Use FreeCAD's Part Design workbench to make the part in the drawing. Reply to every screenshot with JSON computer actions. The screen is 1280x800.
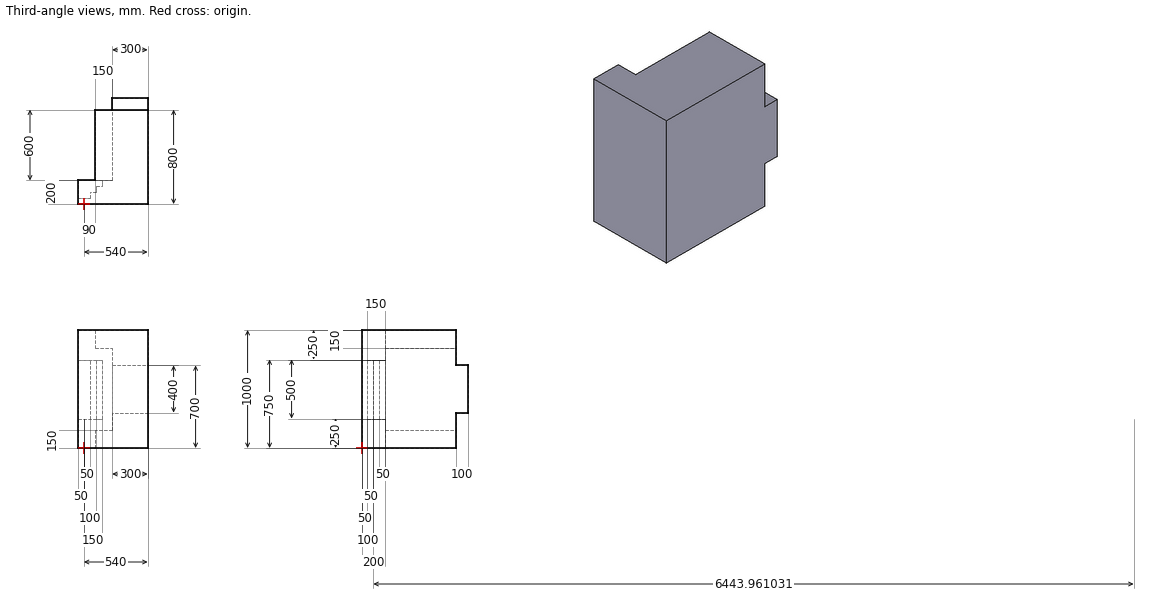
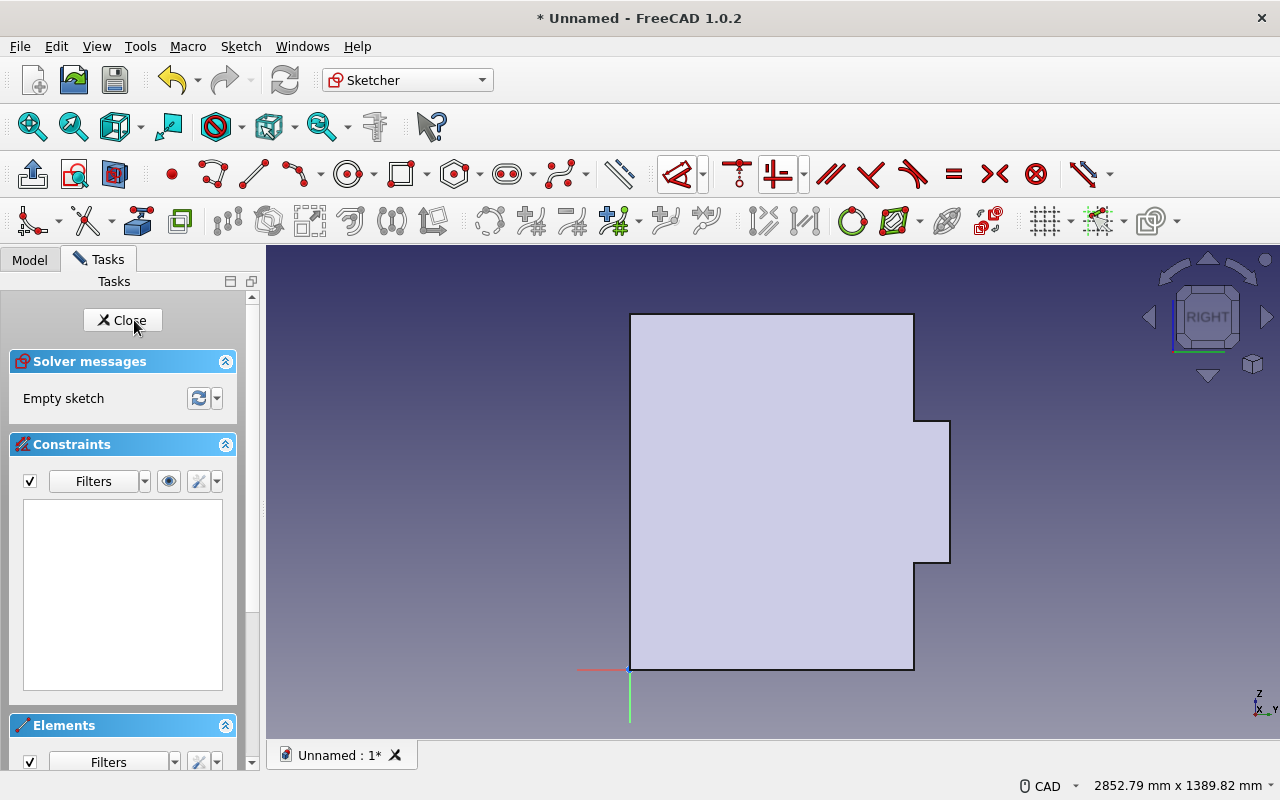
{"action": "left_click", "coordinate": [115, 174]}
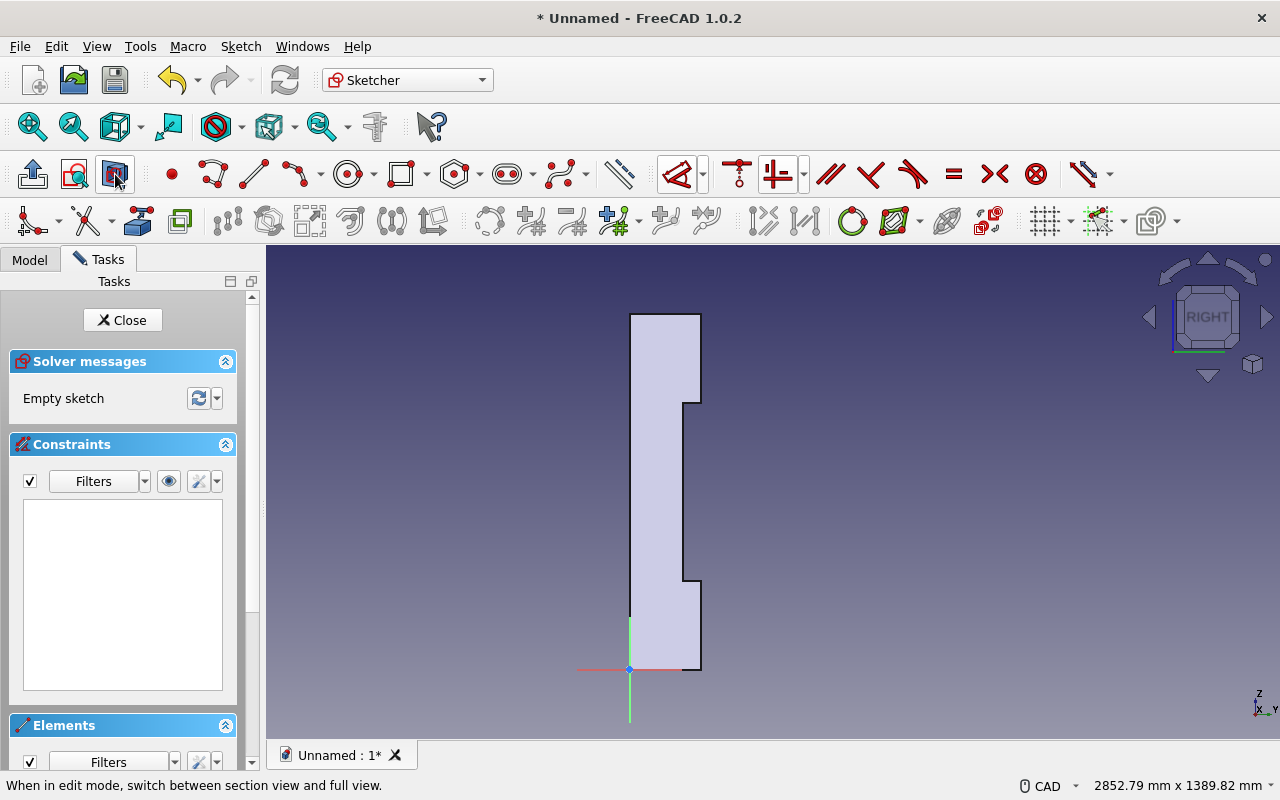
{"action": "scroll", "coordinate": [348, 477], "scroll_direction": "down", "scroll_amount": 7}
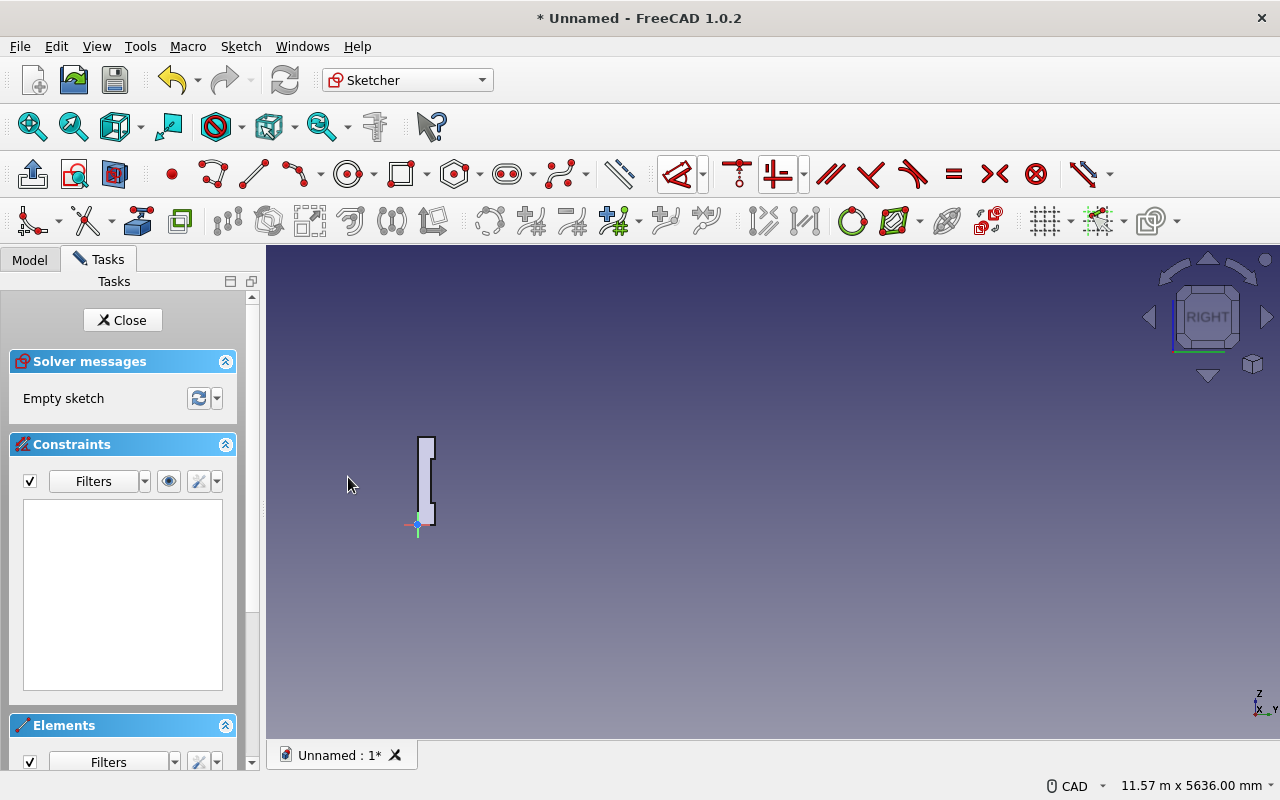
{"action": "left_click", "coordinate": [400, 174]}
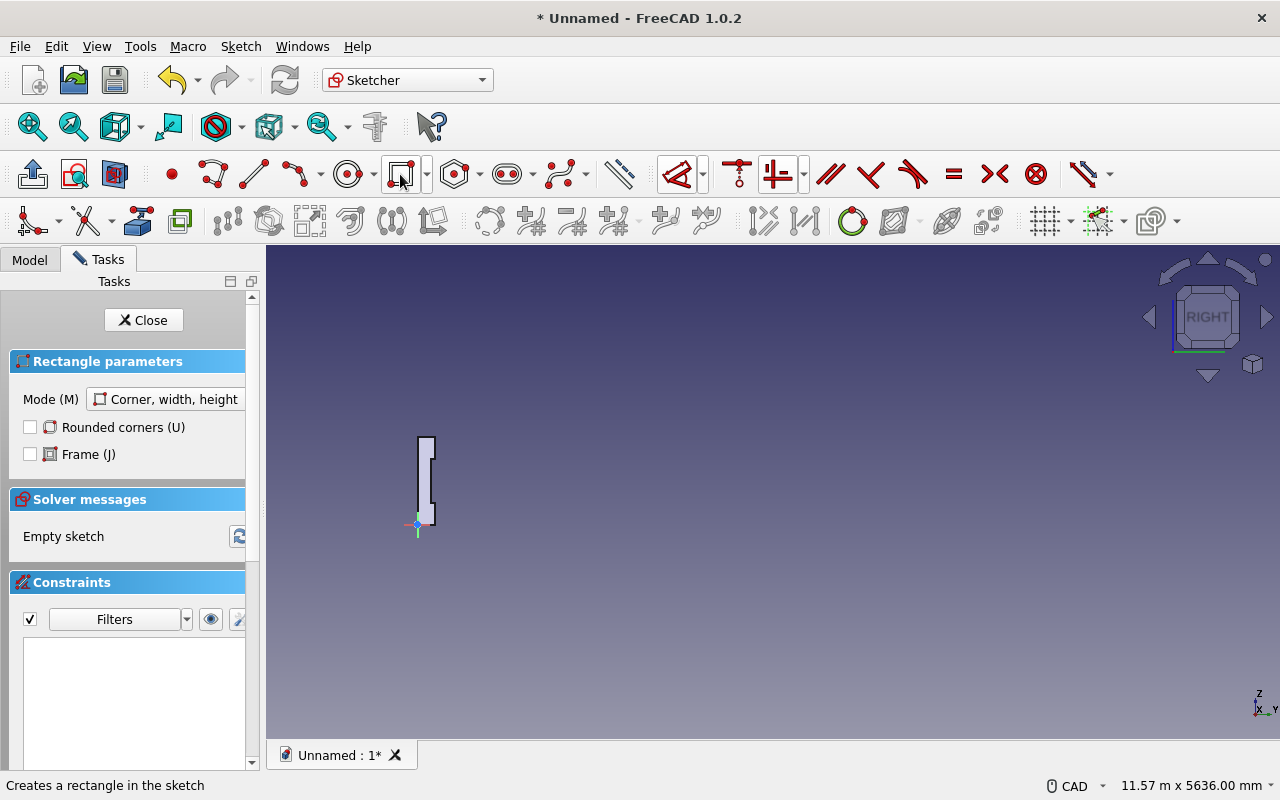
{"action": "scroll", "coordinate": [426, 459], "scroll_direction": "up", "scroll_amount": 3}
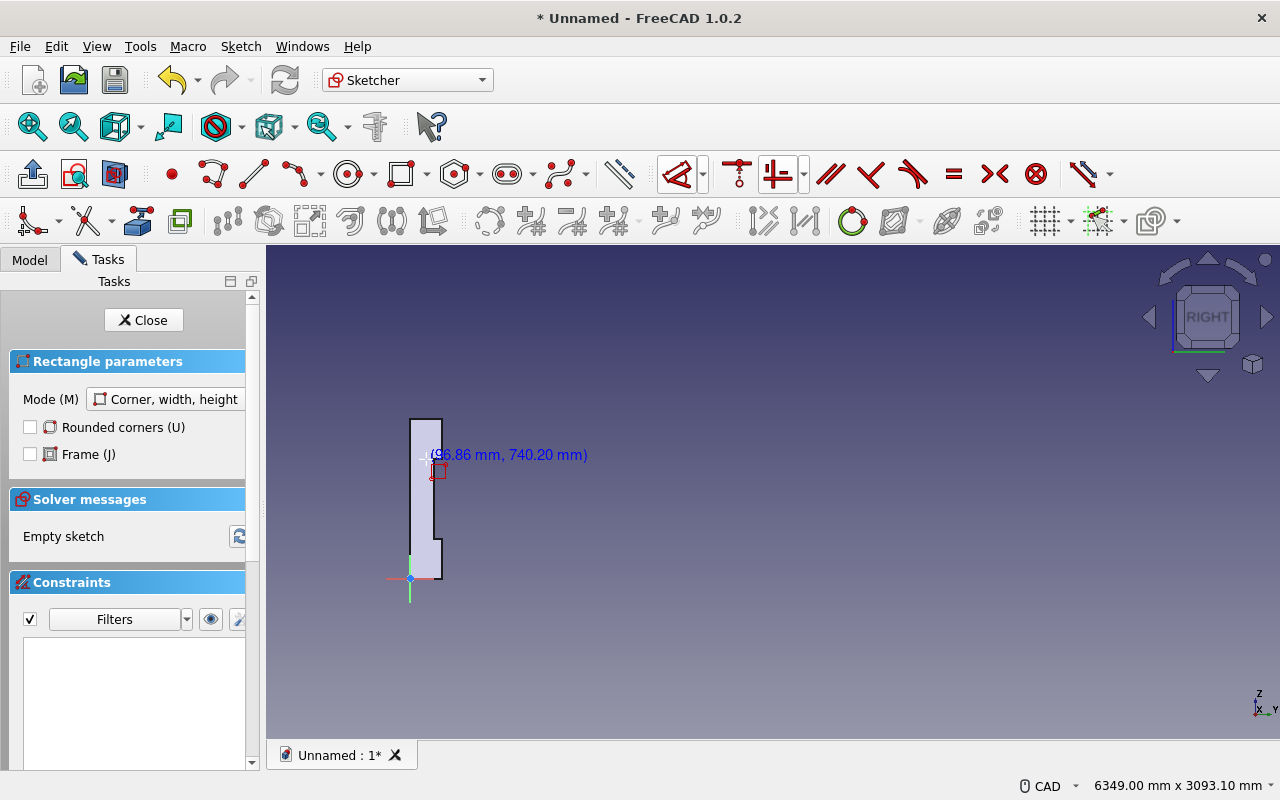
{"action": "left_click", "coordinate": [426, 459]}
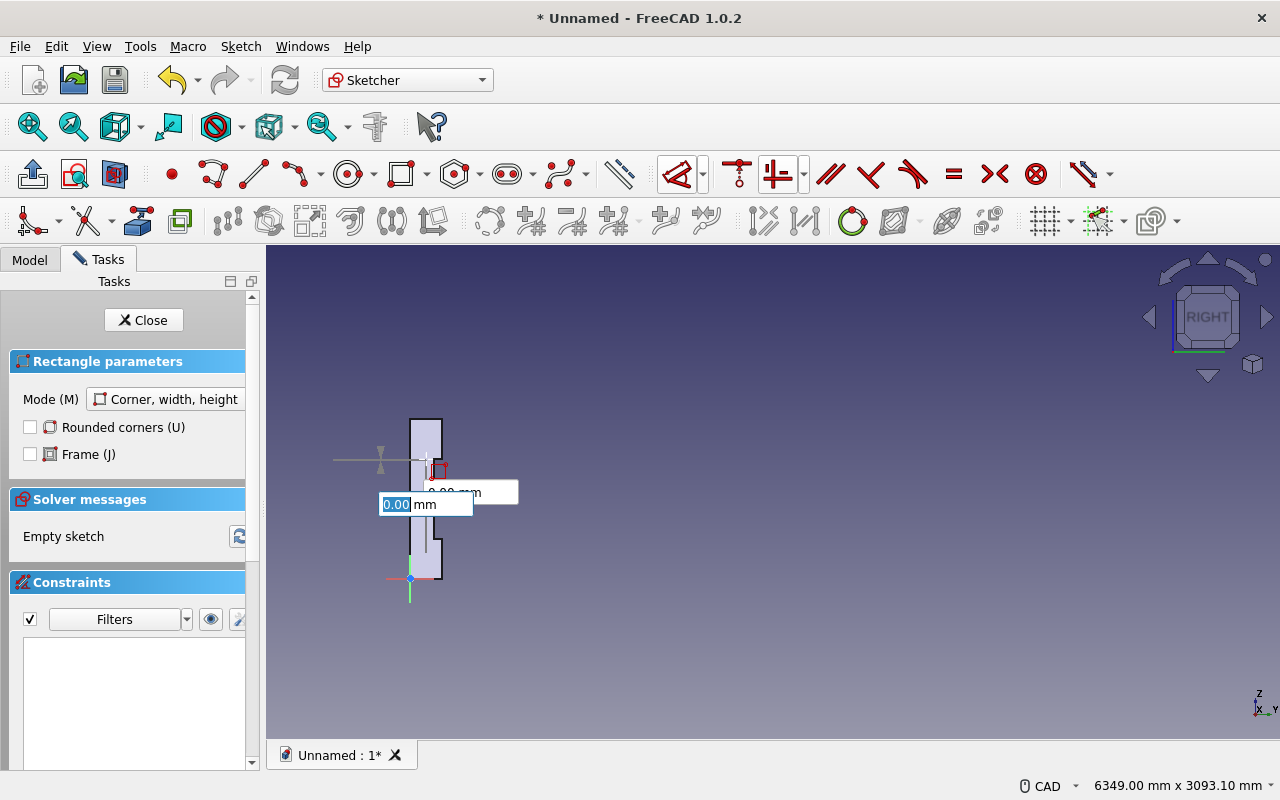
{"action": "scroll", "coordinate": [427, 459], "scroll_direction": "down", "scroll_amount": 3}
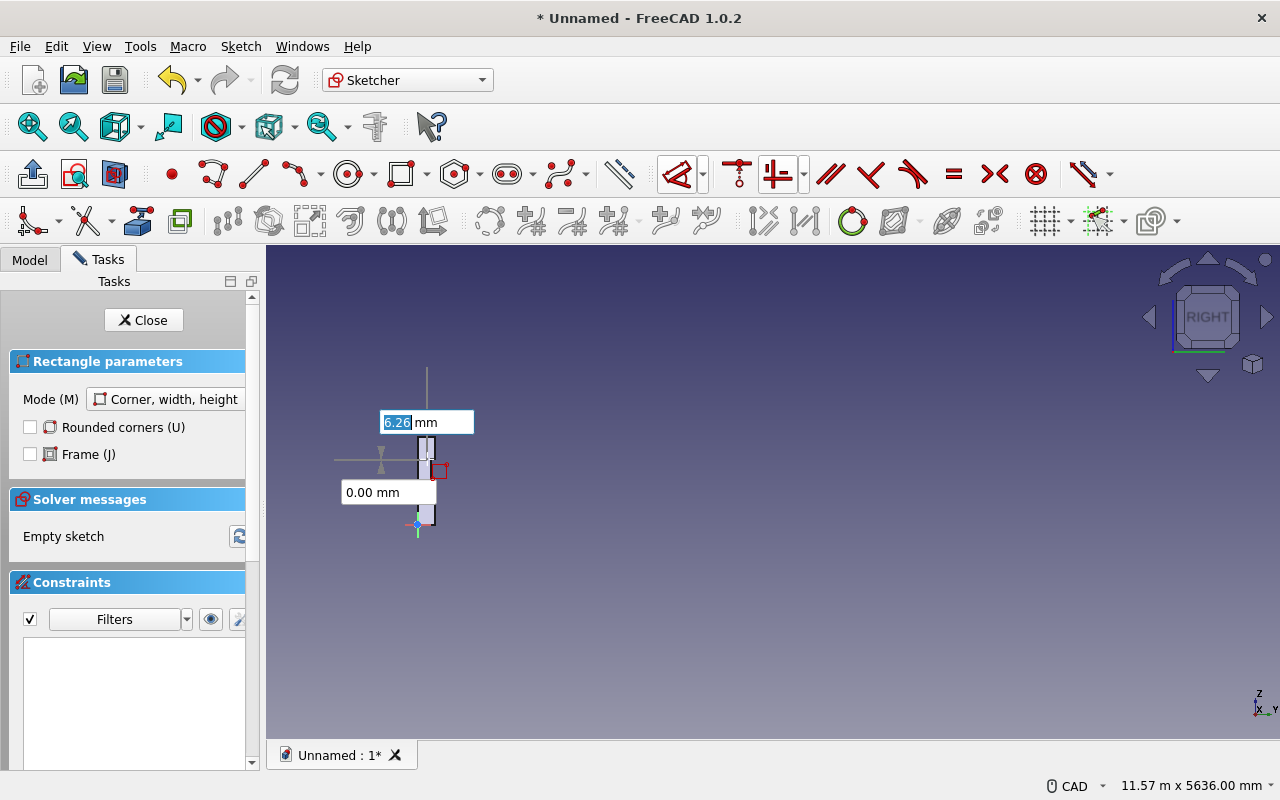
{"action": "left_click", "coordinate": [992, 503]}
{"action": "key", "text": "Escape"}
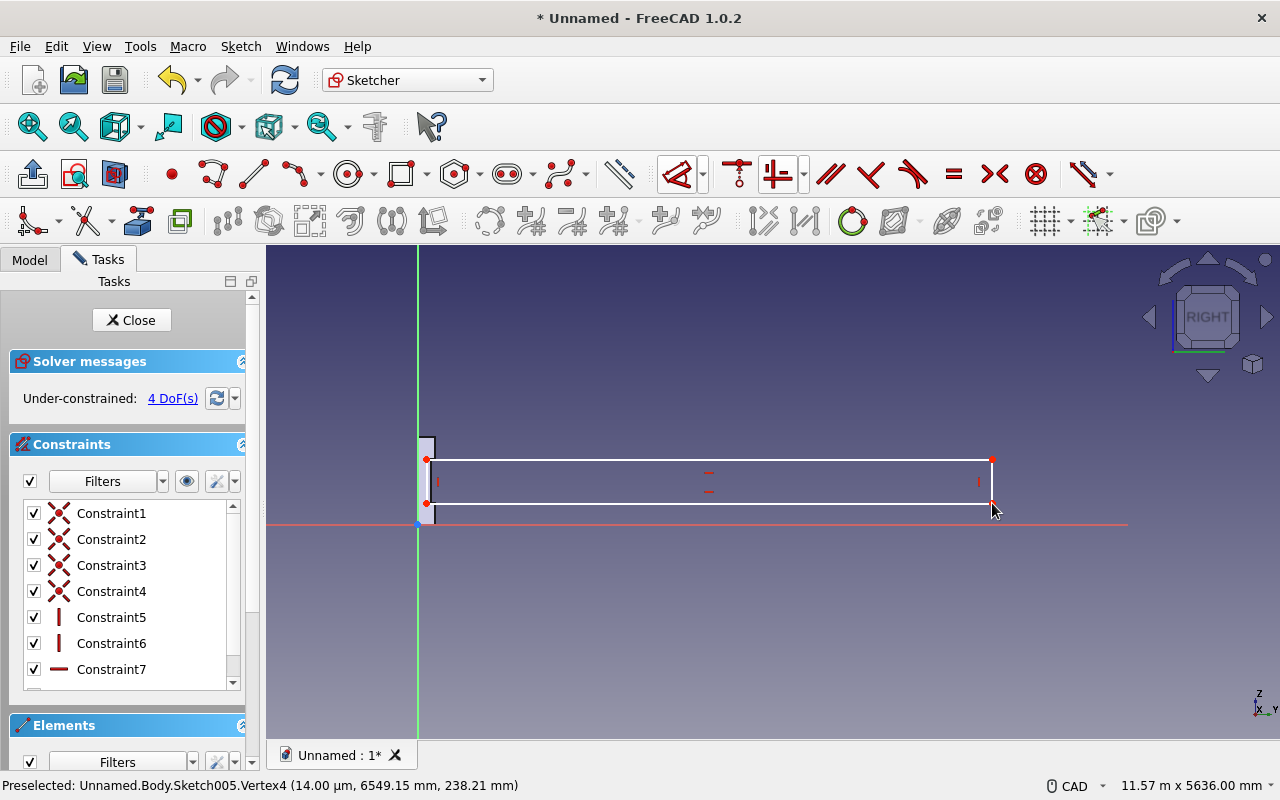
{"action": "scroll", "coordinate": [427, 473], "scroll_direction": "up", "scroll_amount": 3}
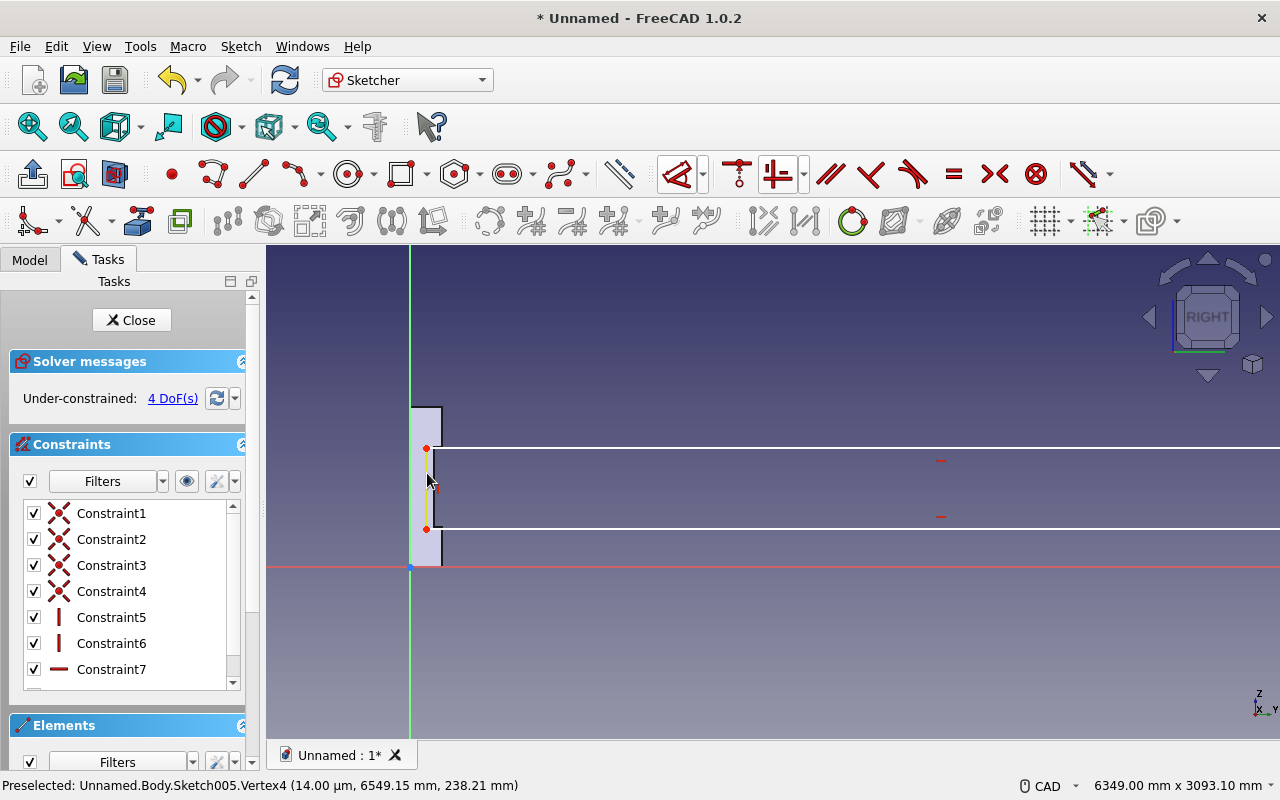
{"action": "left_click", "coordinate": [426, 473]}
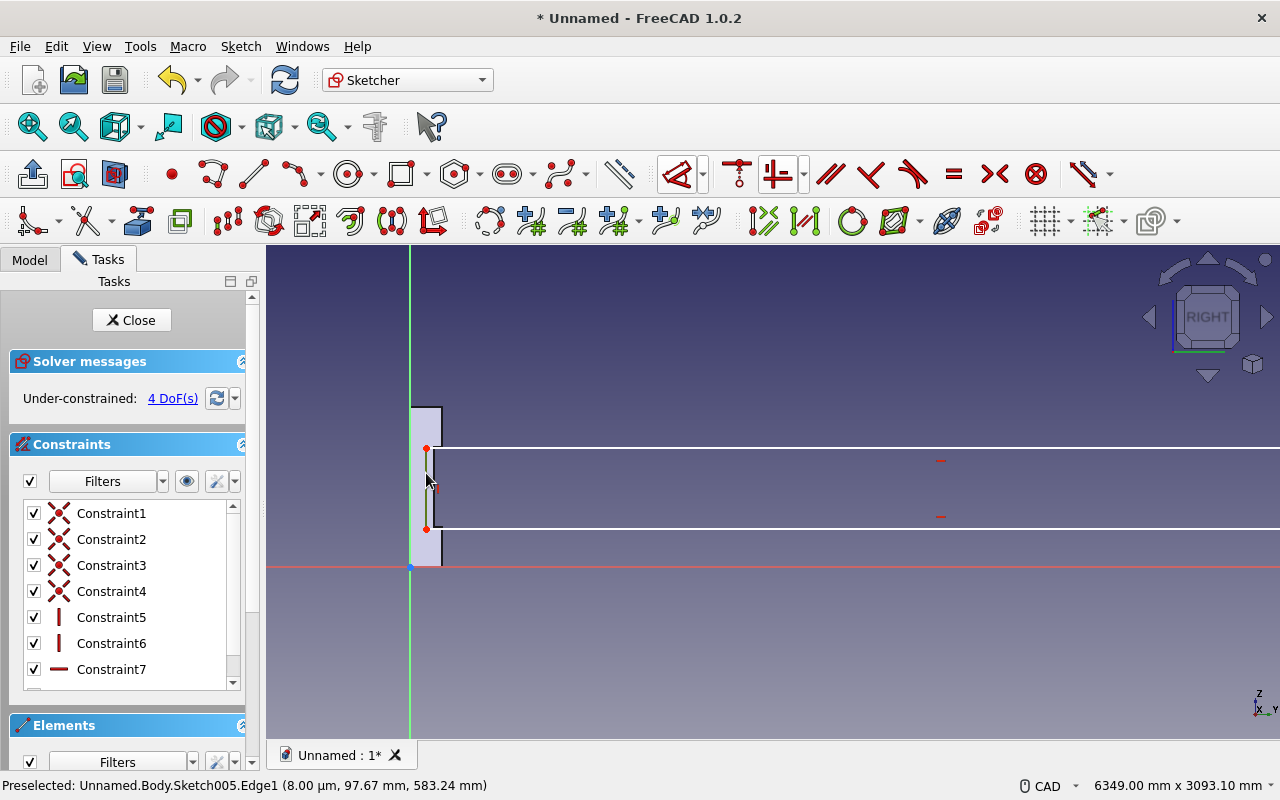
{"action": "left_click", "coordinate": [702, 174]}